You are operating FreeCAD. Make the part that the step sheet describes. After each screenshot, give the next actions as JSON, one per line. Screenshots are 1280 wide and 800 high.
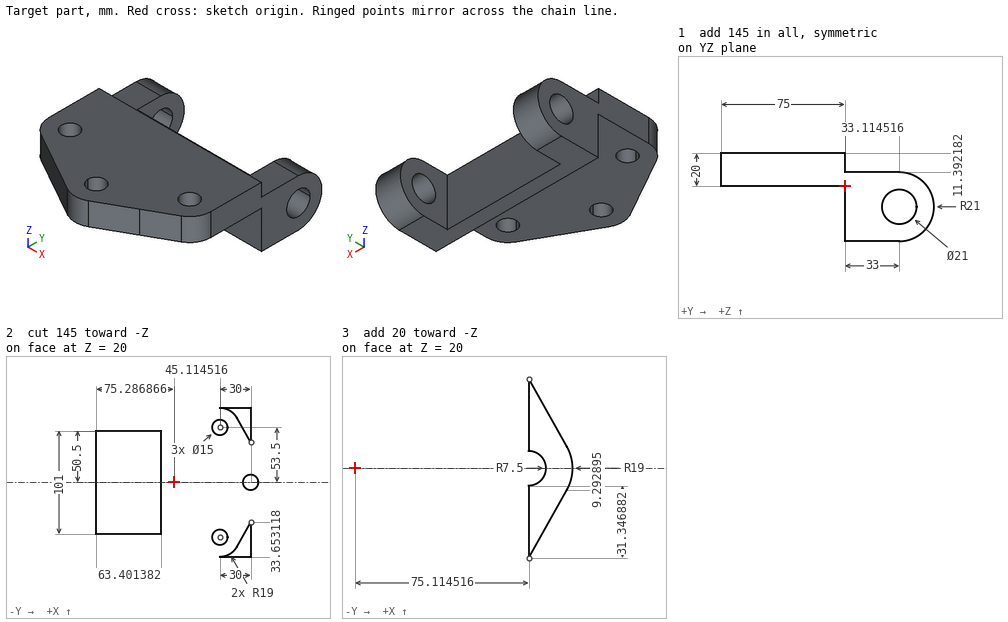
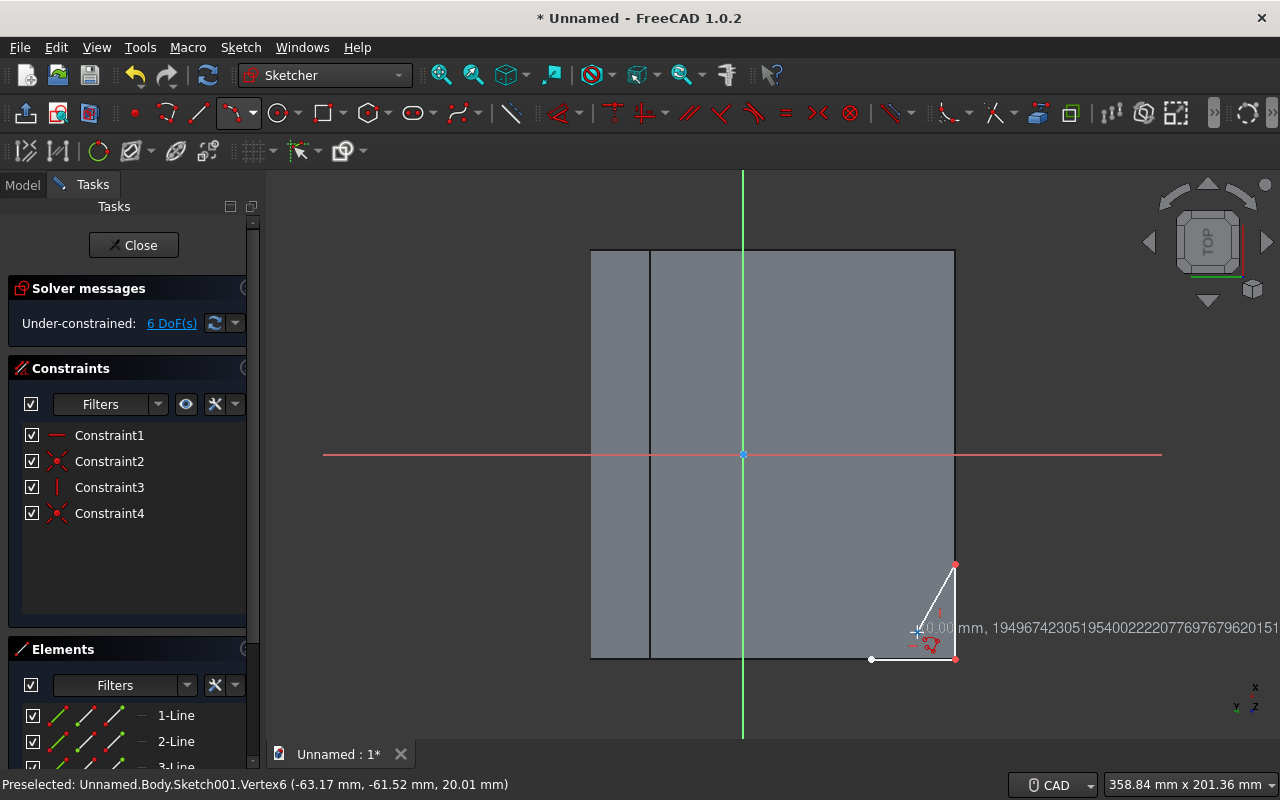
{"action": "left_click", "coordinate": [232, 114]}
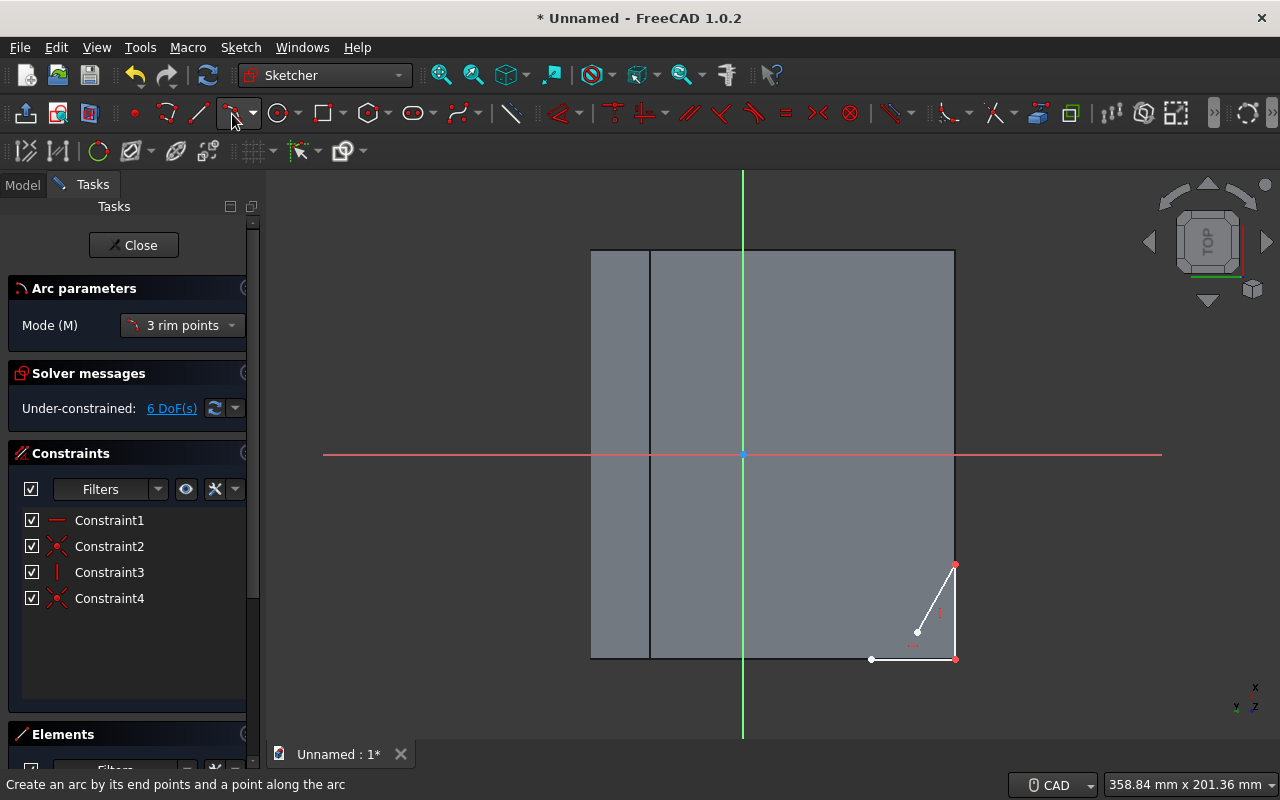
{"action": "left_click", "coordinate": [917, 633]}
{"action": "left_click", "coordinate": [871, 660]}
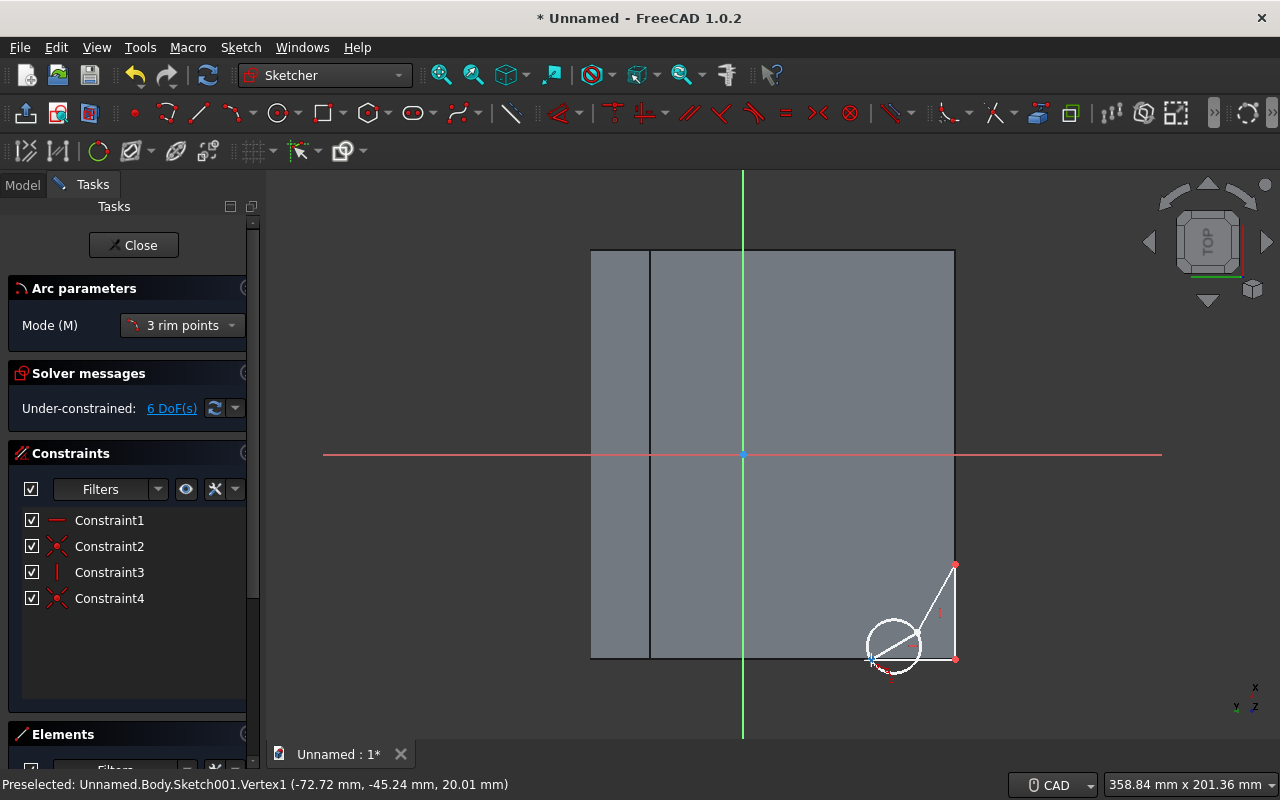
{"action": "scroll", "coordinate": [898, 652], "scroll_direction": "up", "scroll_amount": 4}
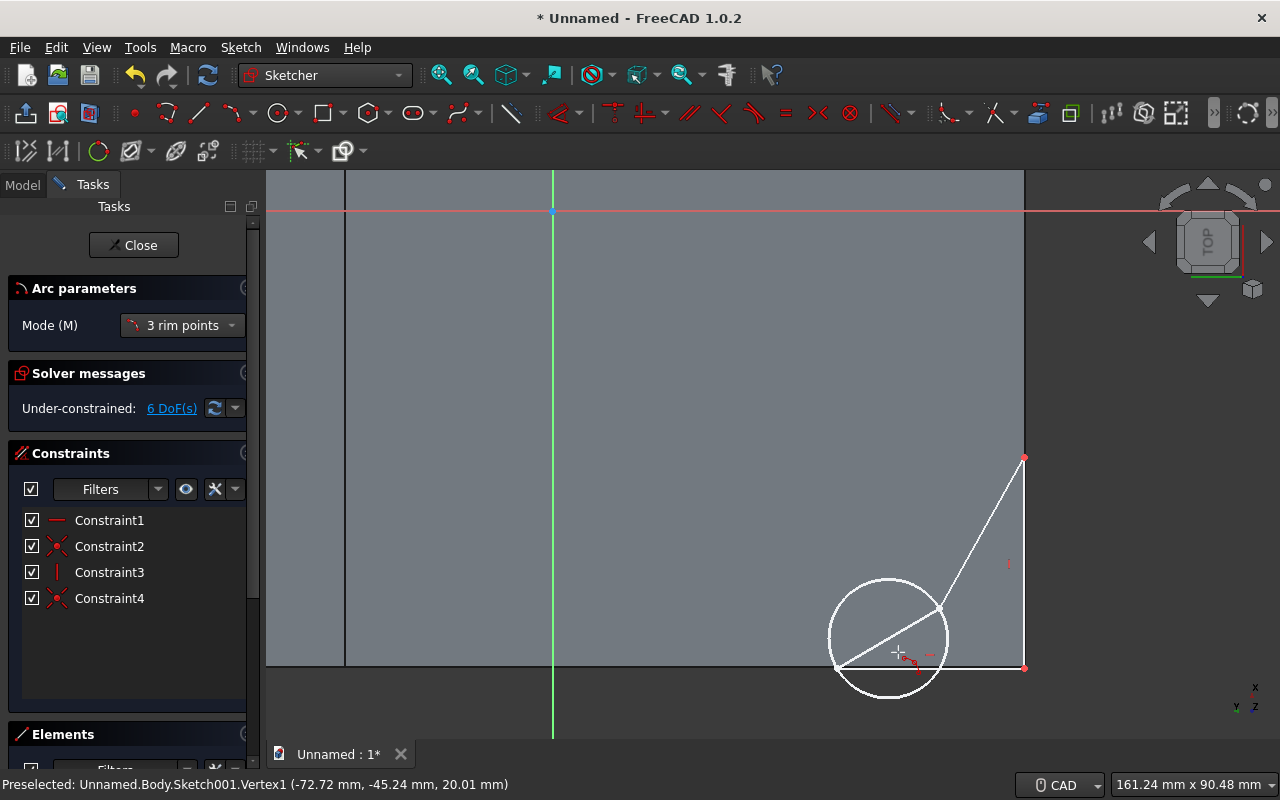
{"action": "left_click", "coordinate": [897, 651]}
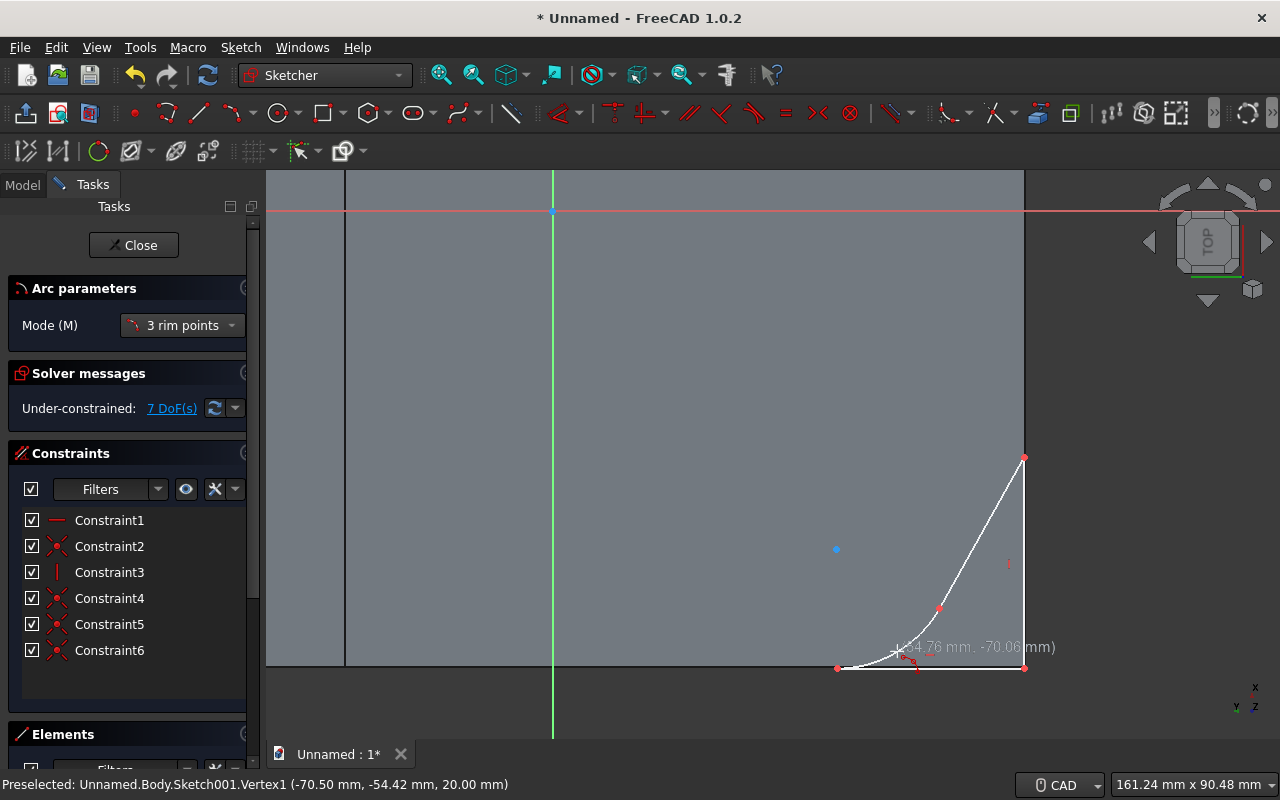
{"action": "left_click", "coordinate": [168, 114]}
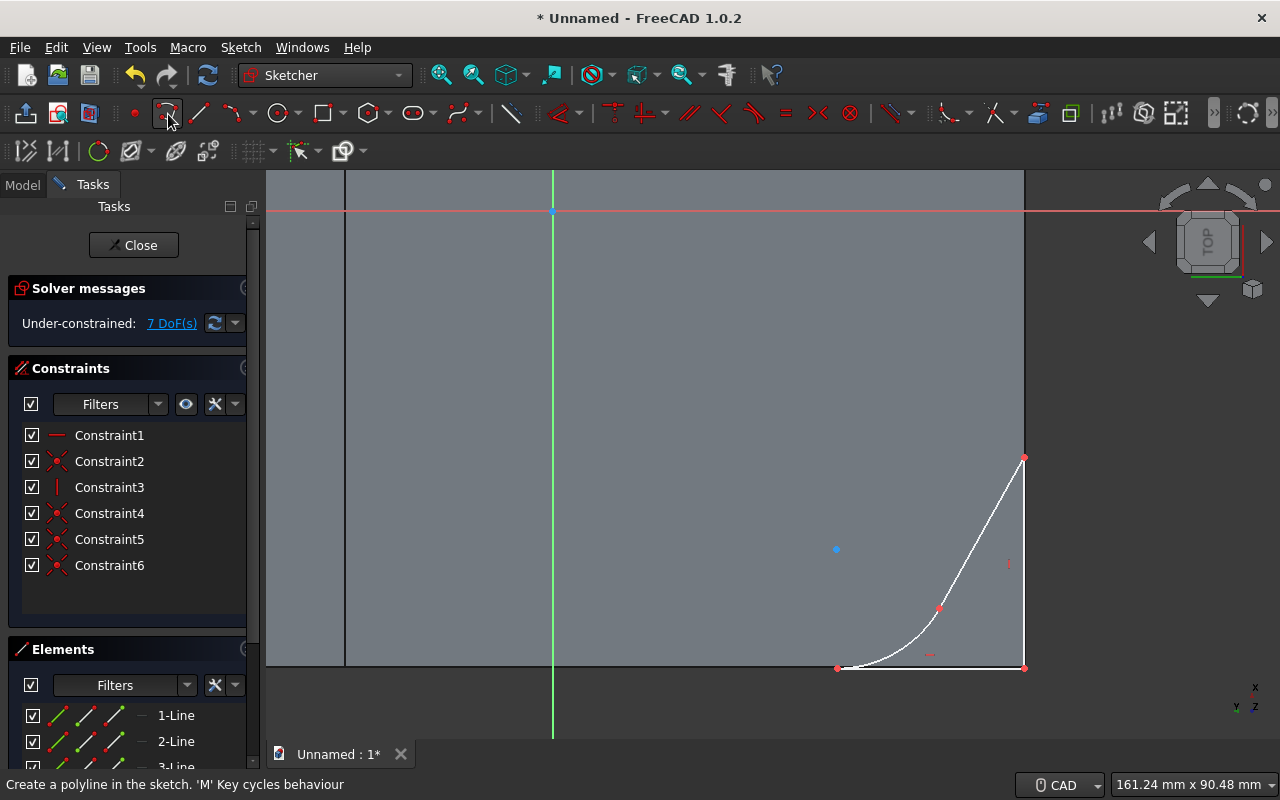
{"action": "scroll", "coordinate": [779, 596], "scroll_direction": "down", "scroll_amount": 5}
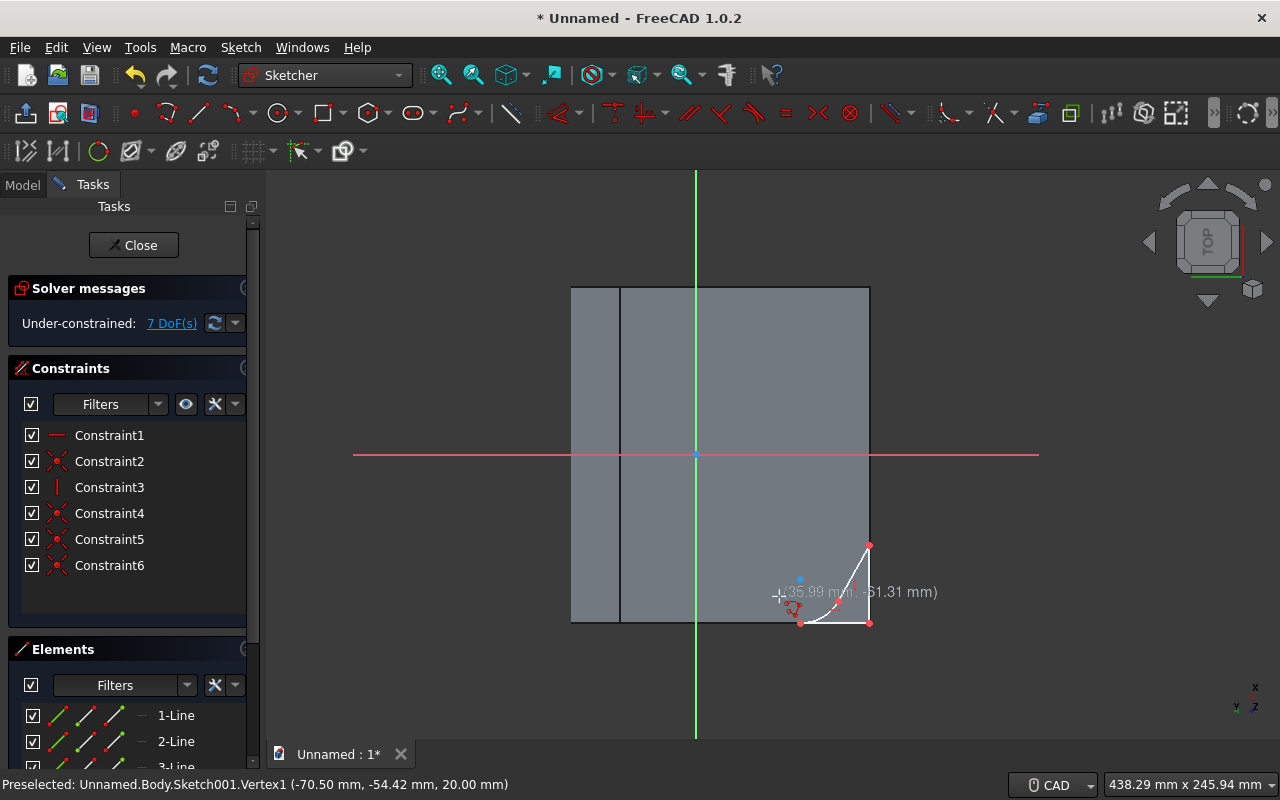
{"action": "left_click", "coordinate": [839, 310]}
{"action": "left_click", "coordinate": [870, 365]}
{"action": "left_click", "coordinate": [870, 287]}
{"action": "left_click", "coordinate": [800, 287]}
{"action": "right_click", "coordinate": [800, 287]}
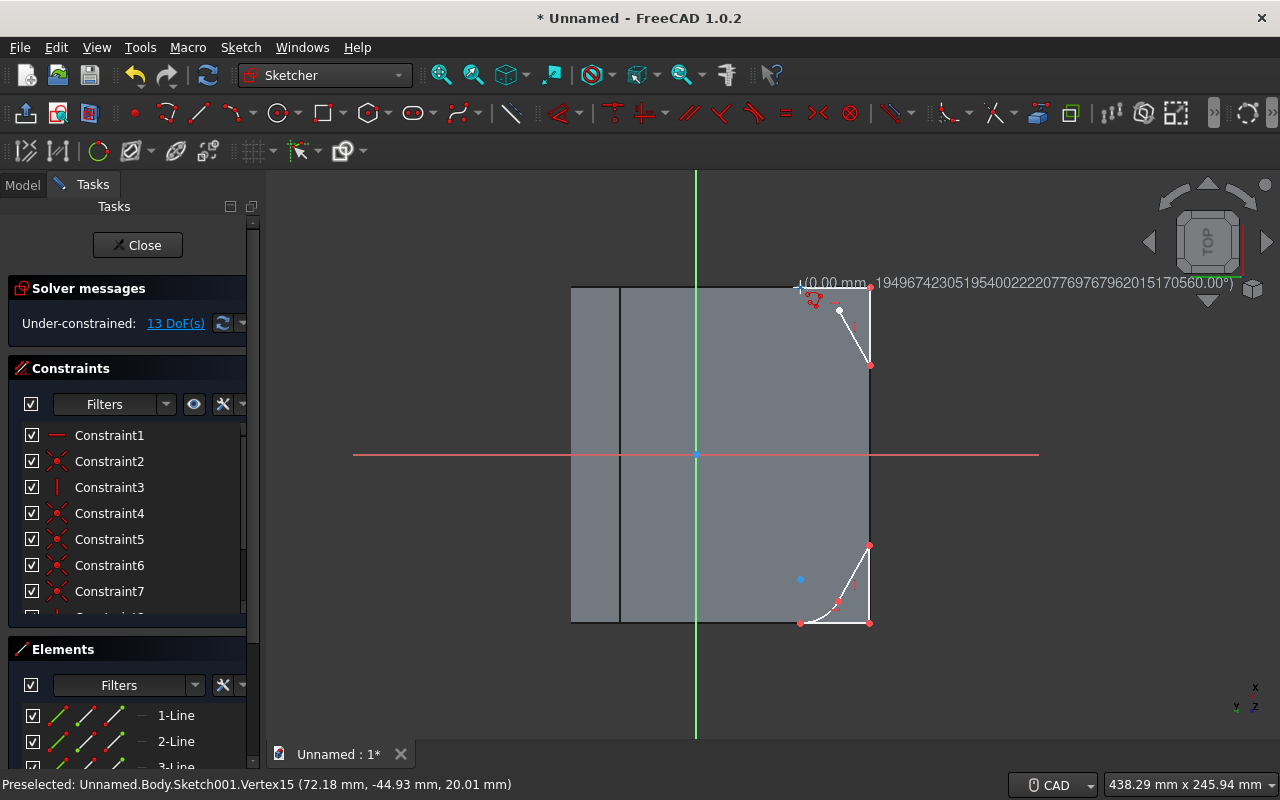
{"action": "left_click", "coordinate": [232, 114]}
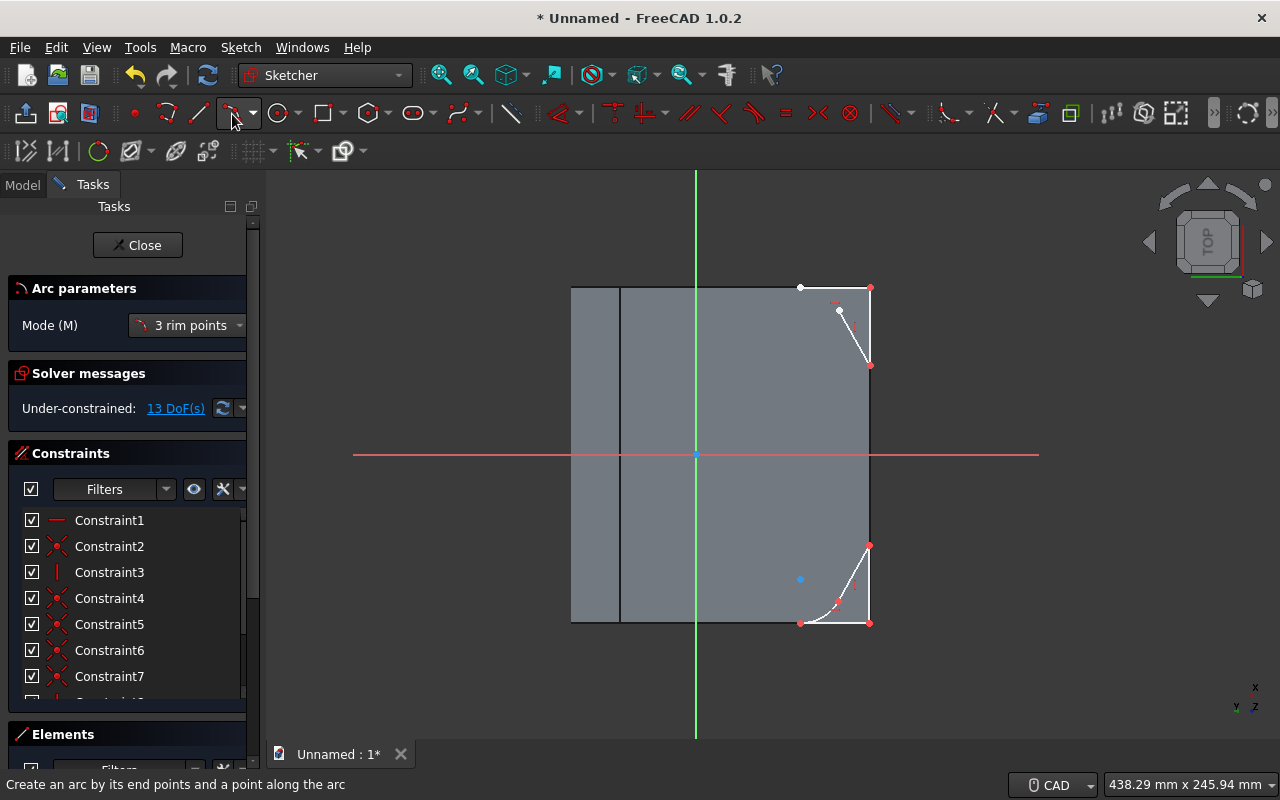
{"action": "left_click", "coordinate": [800, 288]}
{"action": "left_click", "coordinate": [839, 311]}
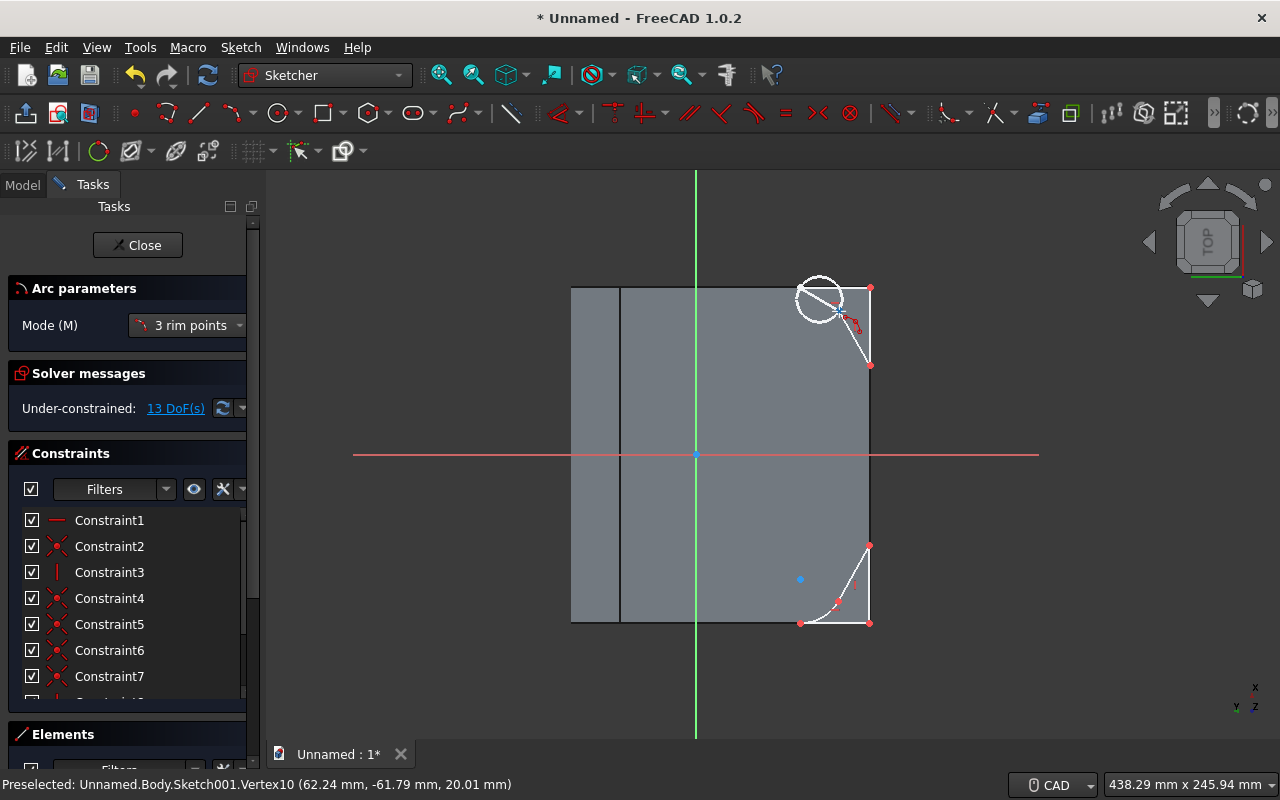
{"action": "scroll", "coordinate": [823, 293], "scroll_direction": "up", "scroll_amount": 5}